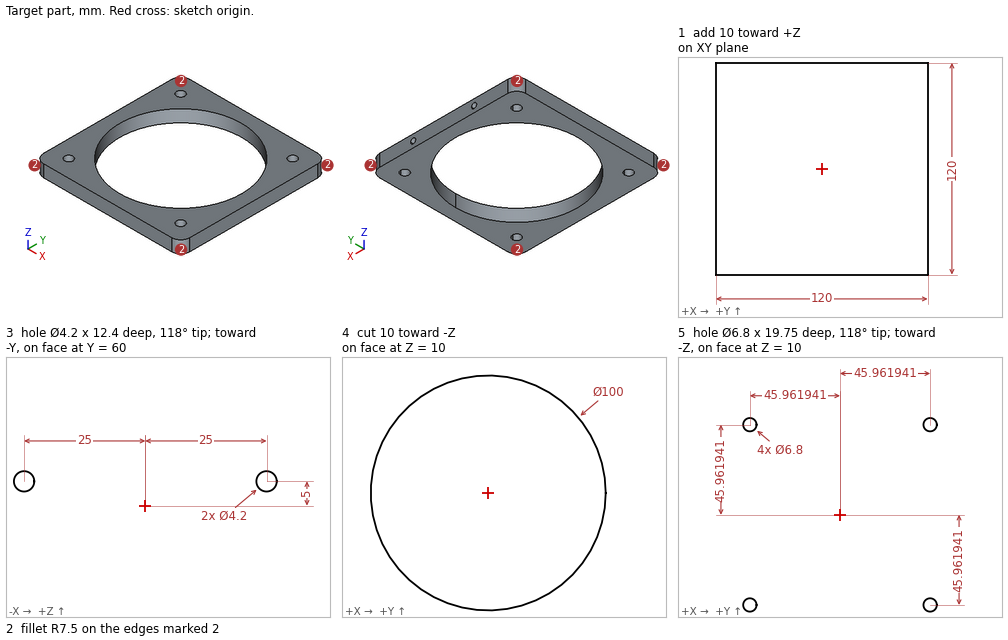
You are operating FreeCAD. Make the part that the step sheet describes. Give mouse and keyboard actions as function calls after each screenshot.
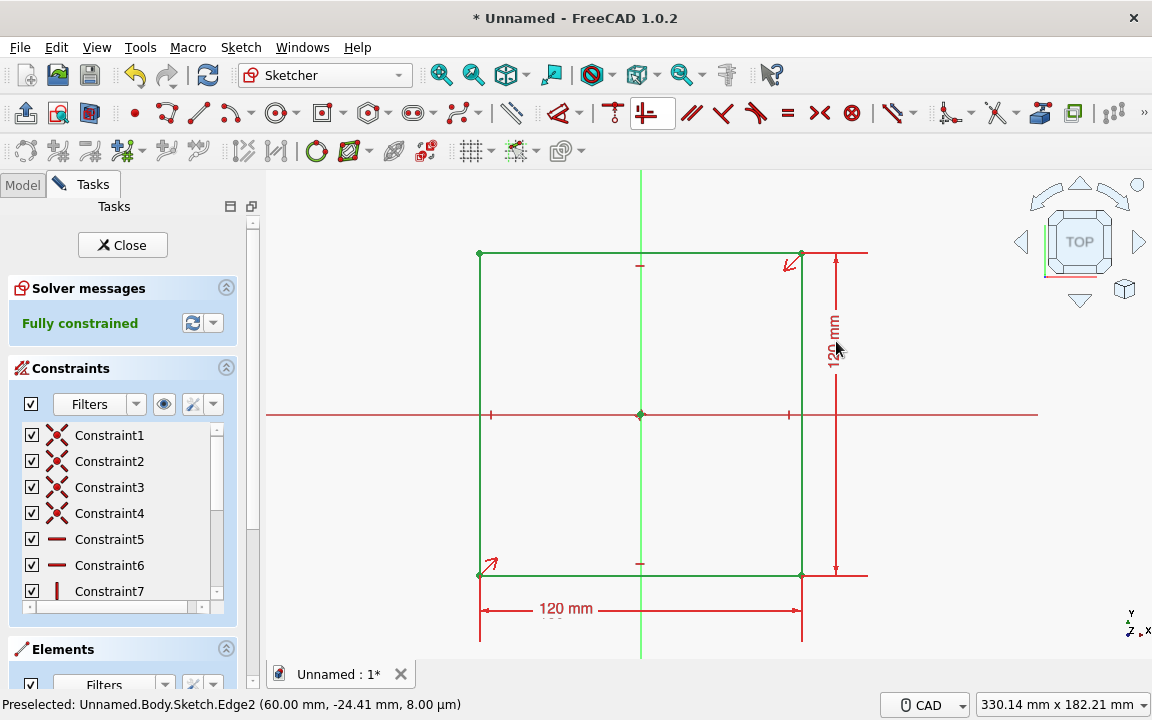
click(123, 245)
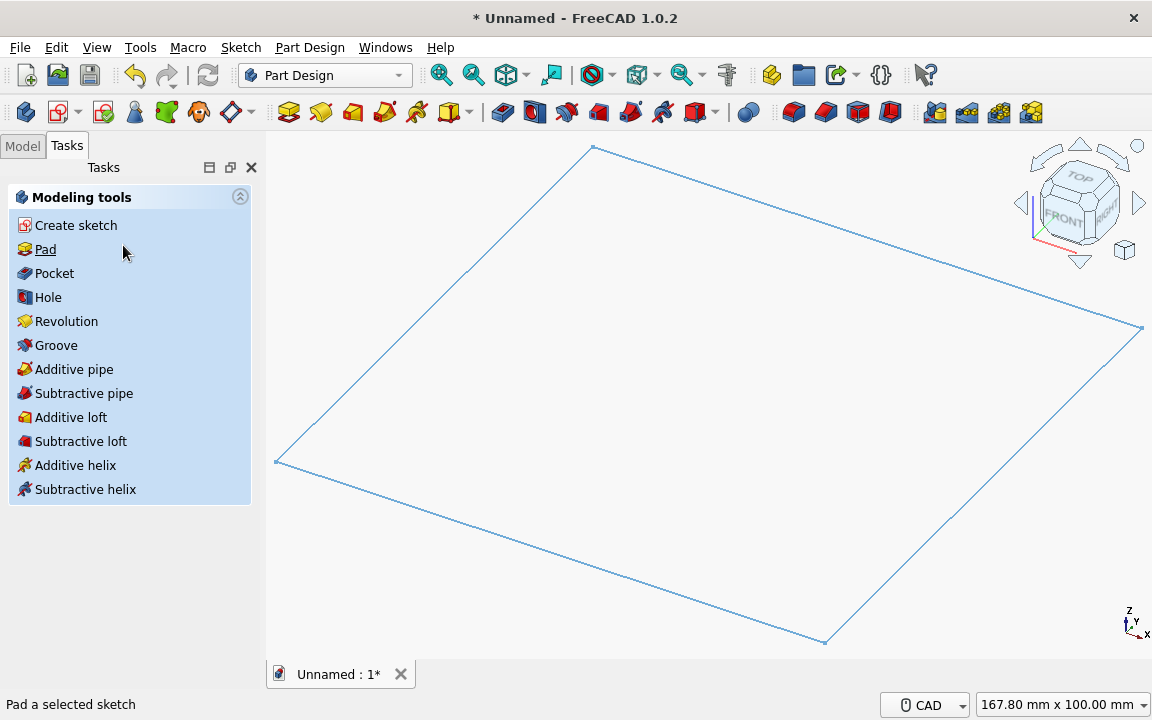
click(290, 112)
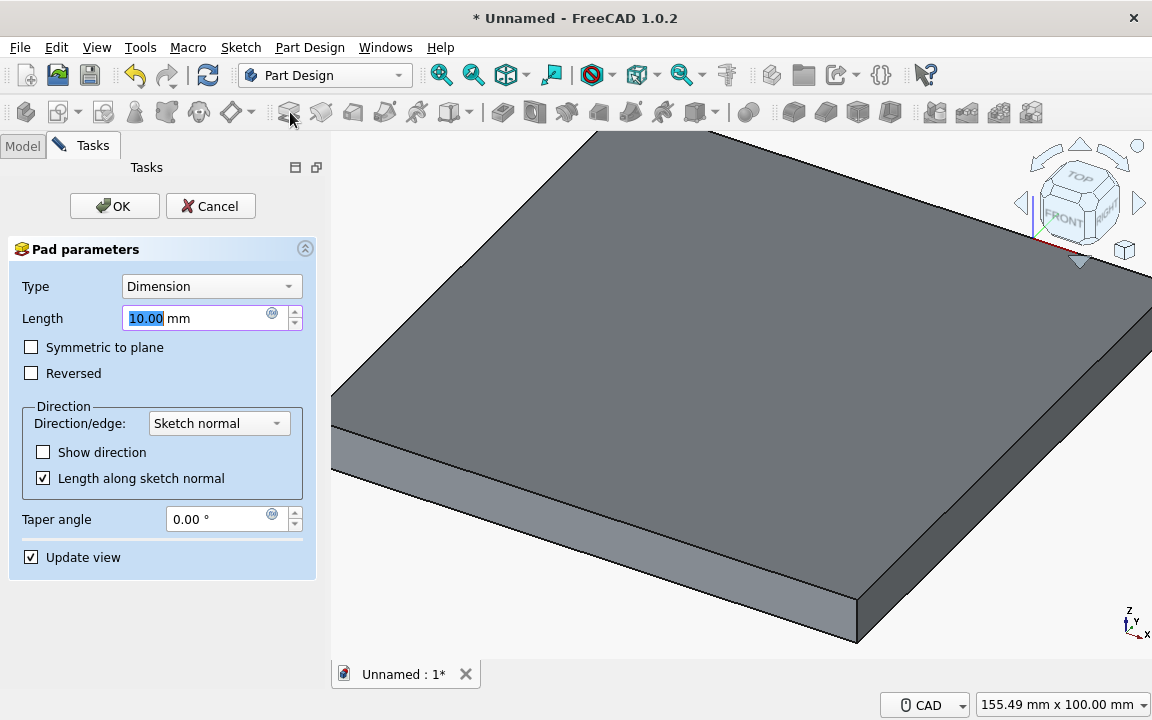
text(10)
key(Tab)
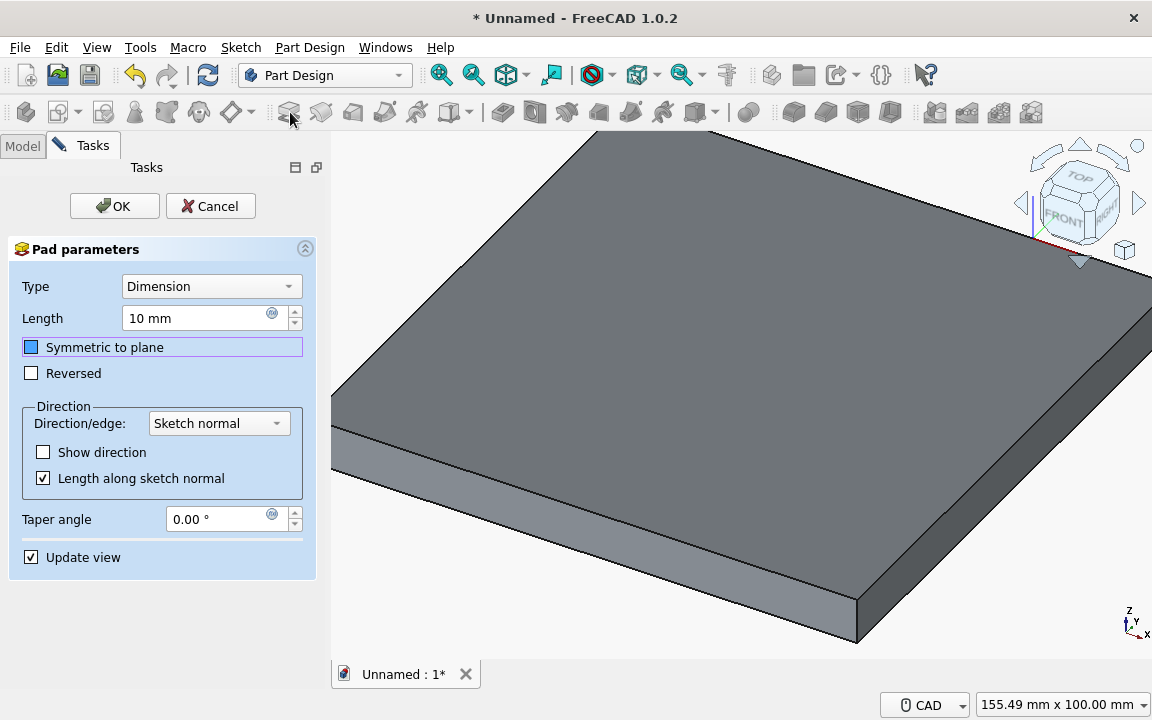
click(115, 206)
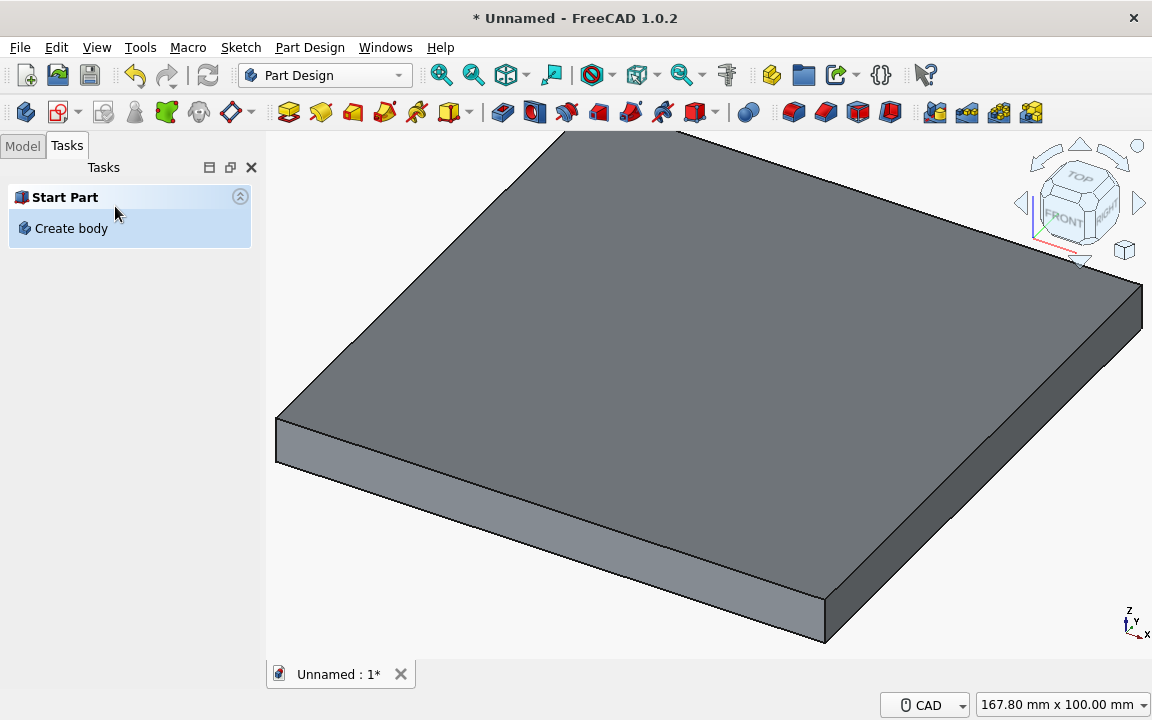
click(442, 76)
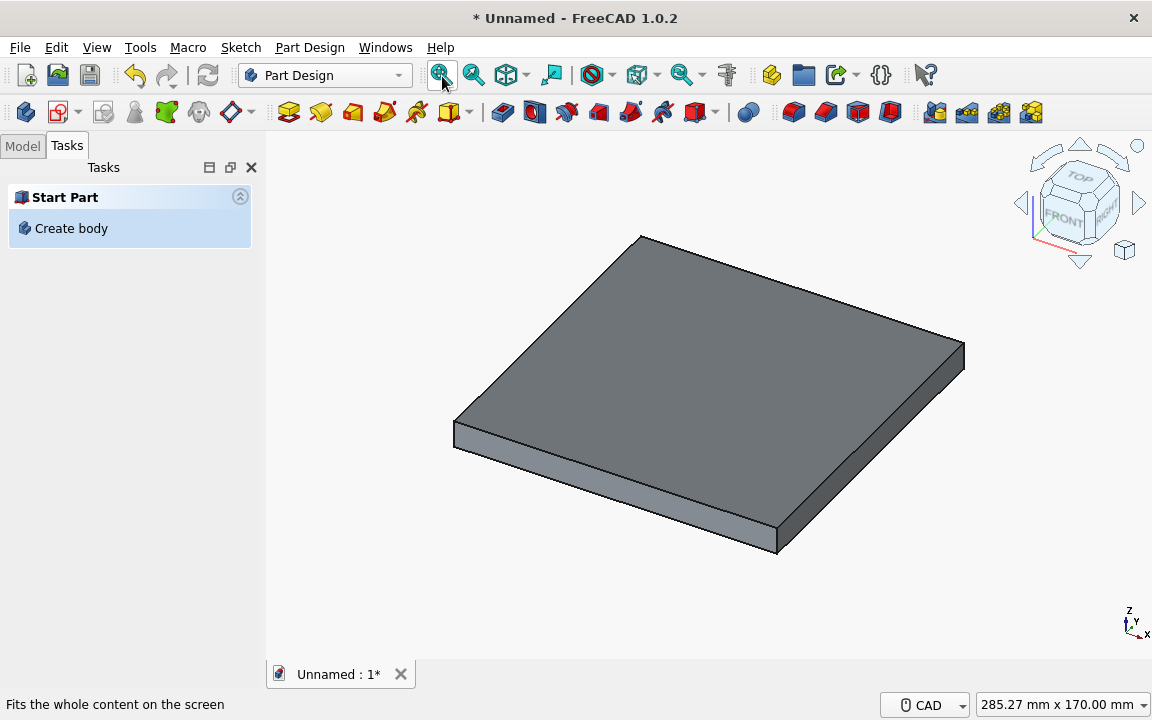
click(777, 540)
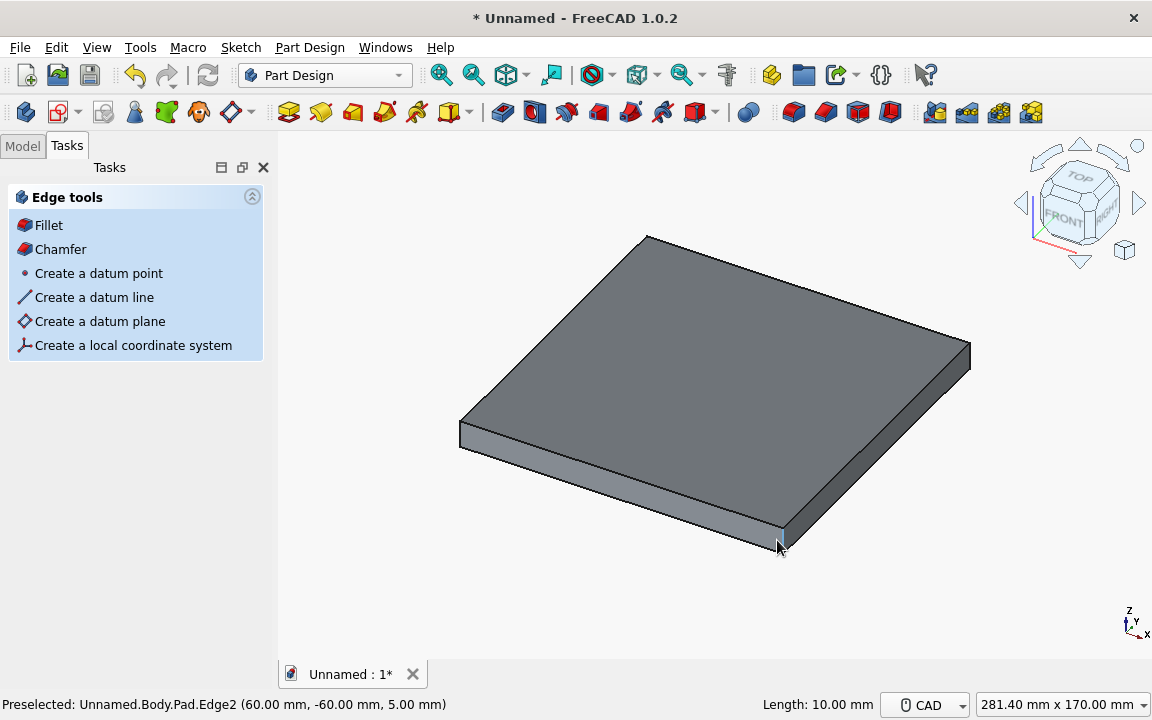
key(0)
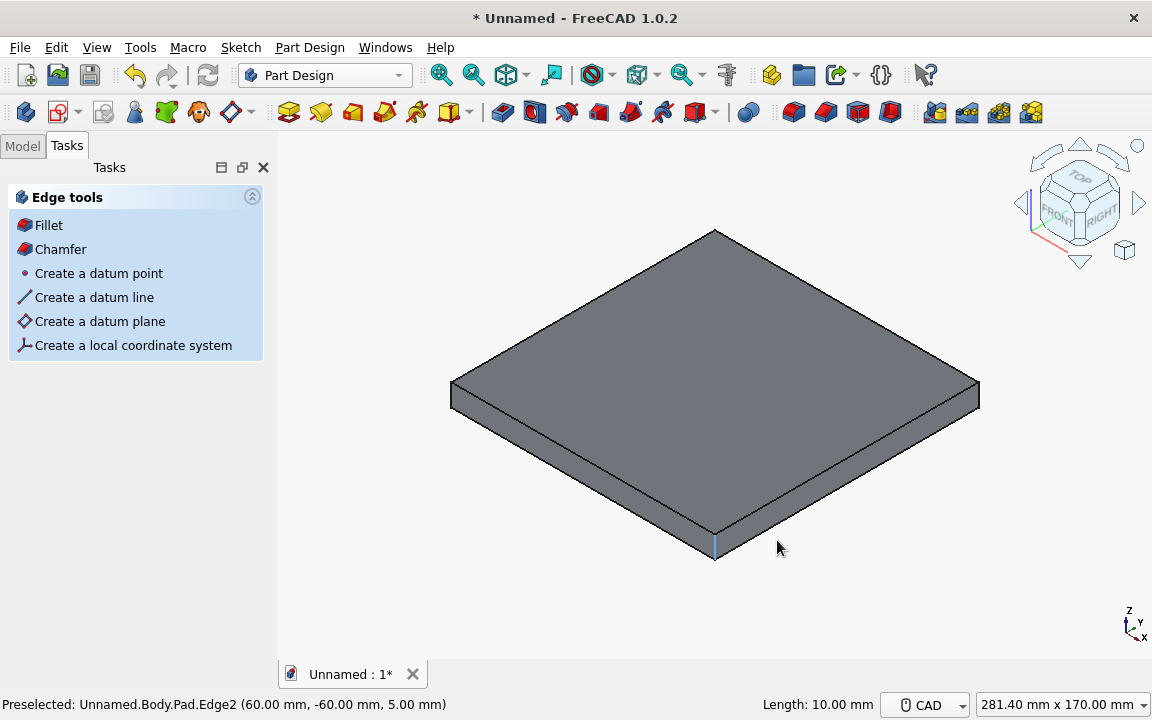
key(2)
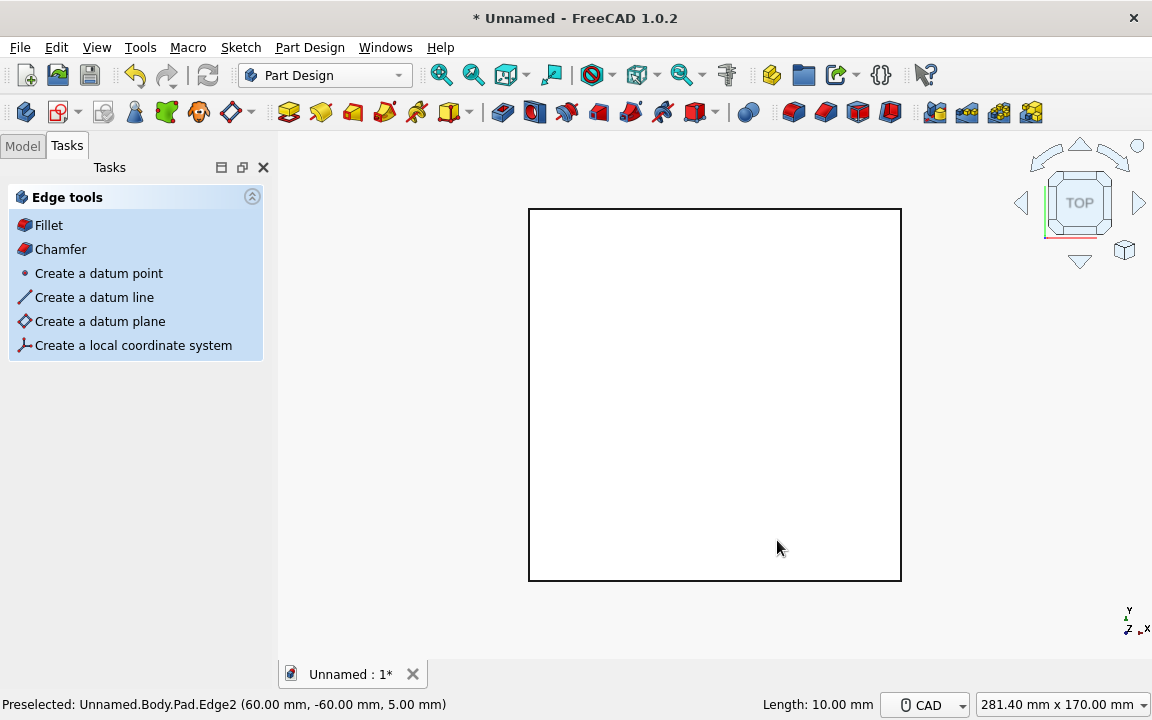
key(1)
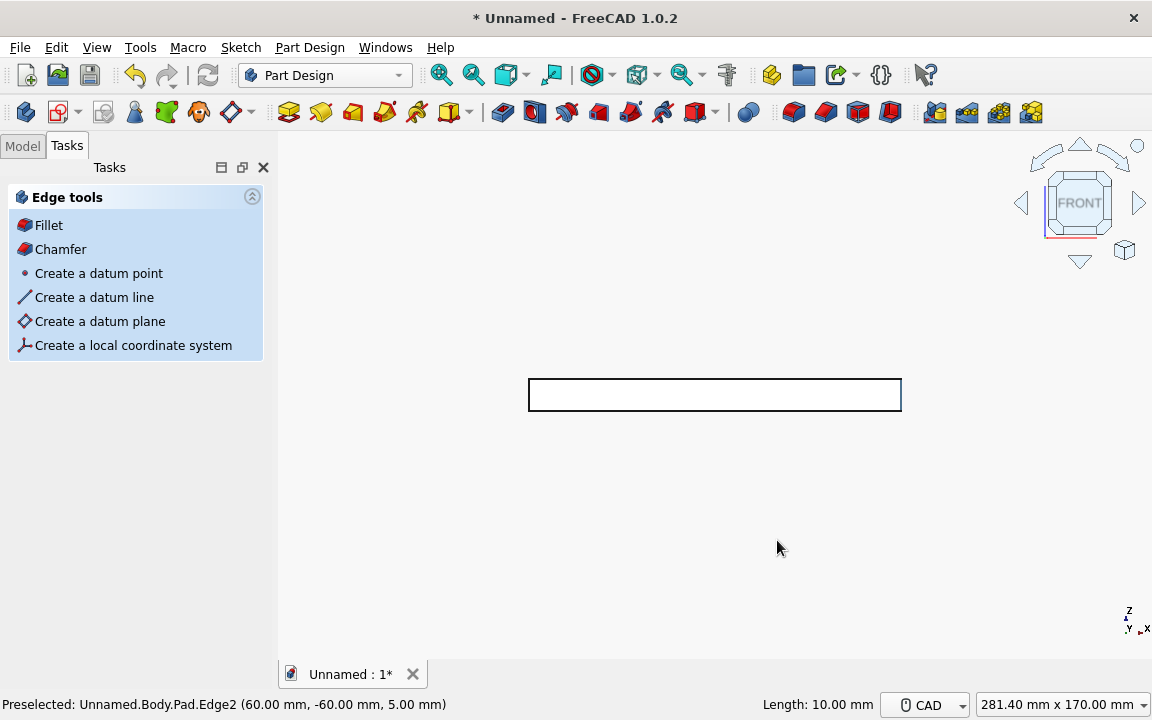
click(442, 76)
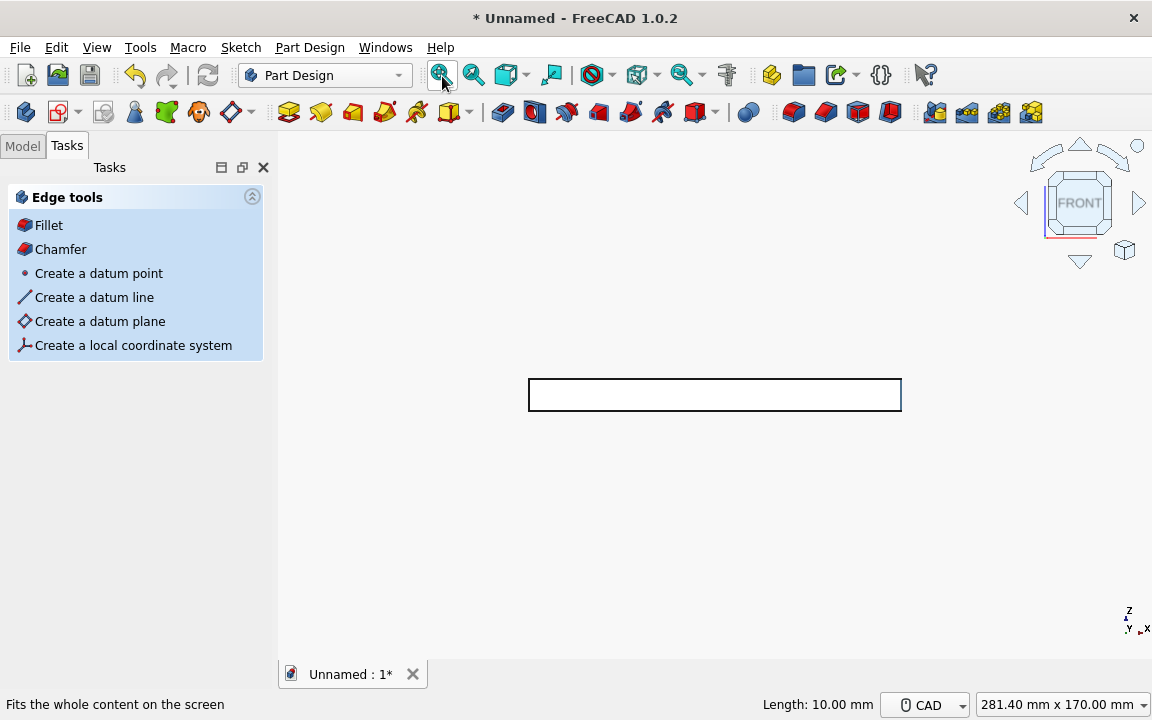
click(529, 394, ctrl)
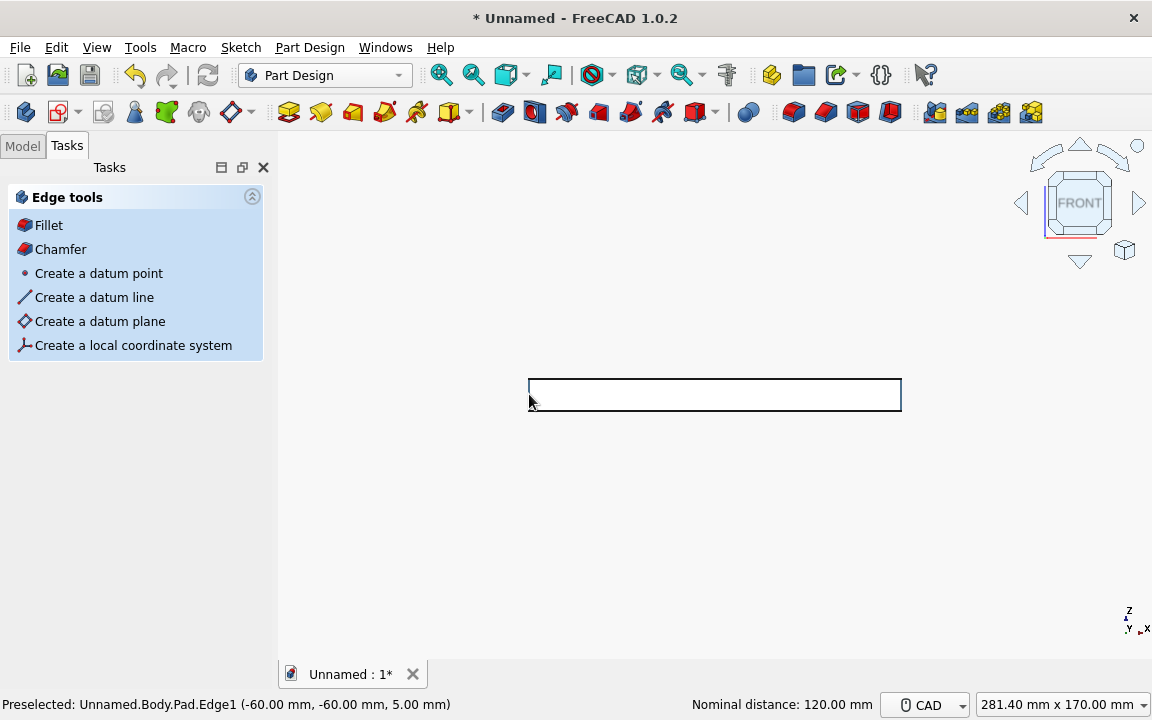
key(3)